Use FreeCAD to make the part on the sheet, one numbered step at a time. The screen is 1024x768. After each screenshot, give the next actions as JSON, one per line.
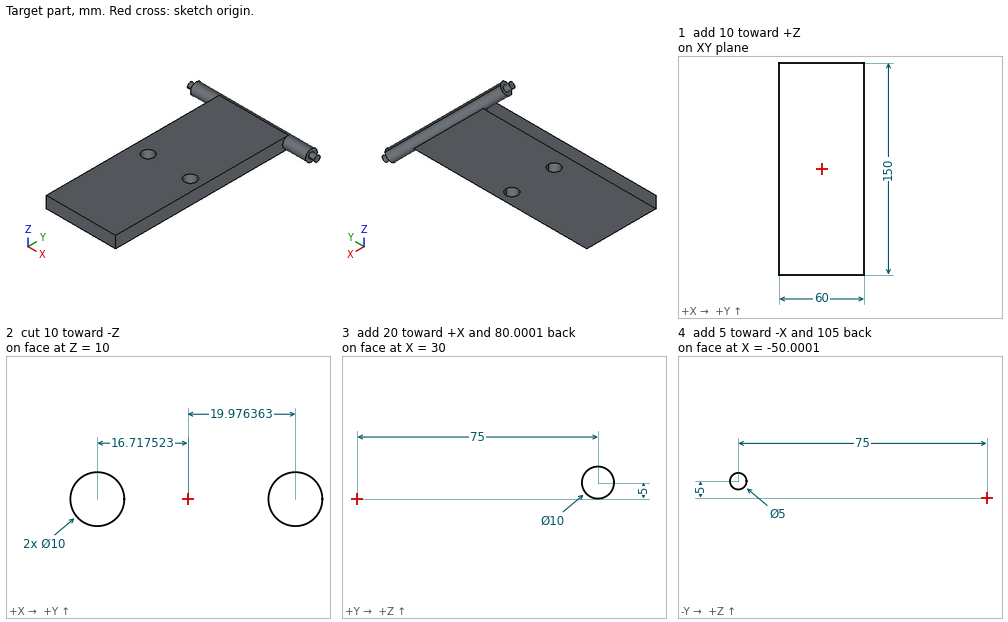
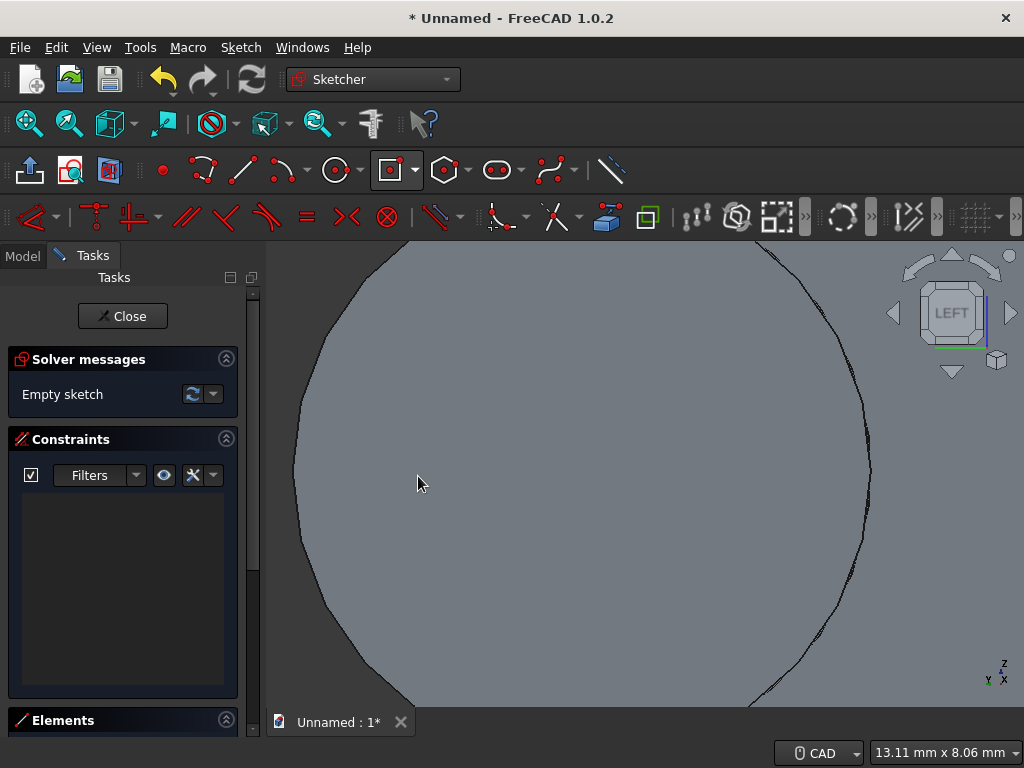
{"action": "left_click", "coordinate": [336, 170]}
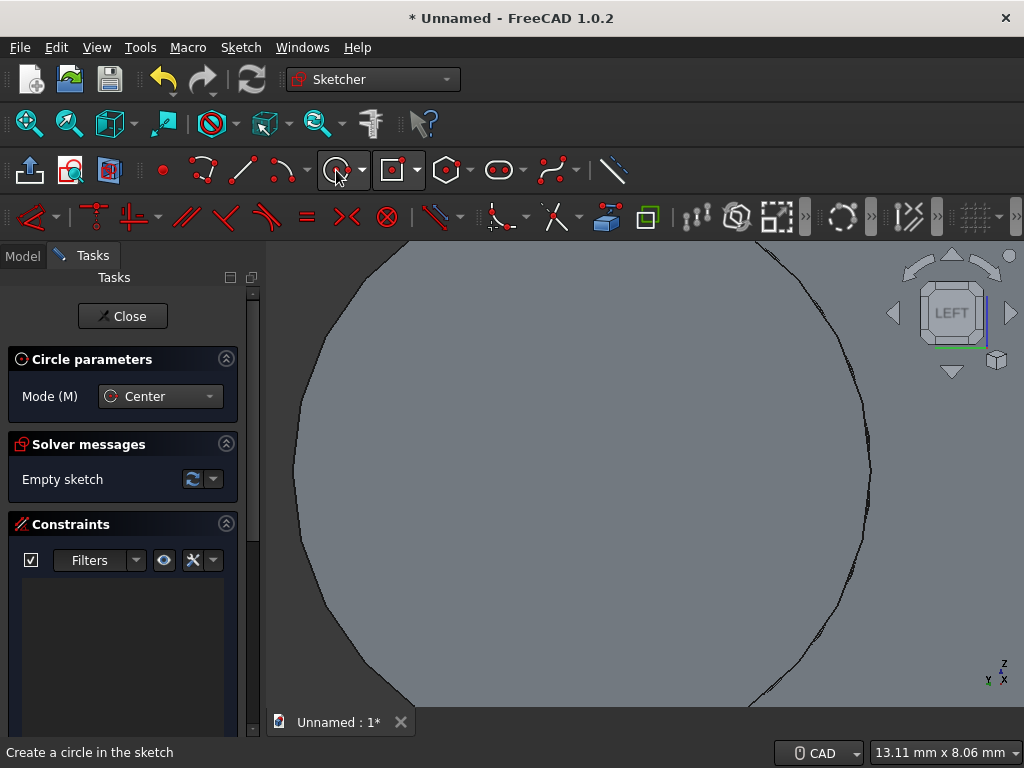
{"action": "left_click", "coordinate": [582, 471]}
{"action": "left_click", "coordinate": [684, 369]}
{"action": "key", "text": "Escape"}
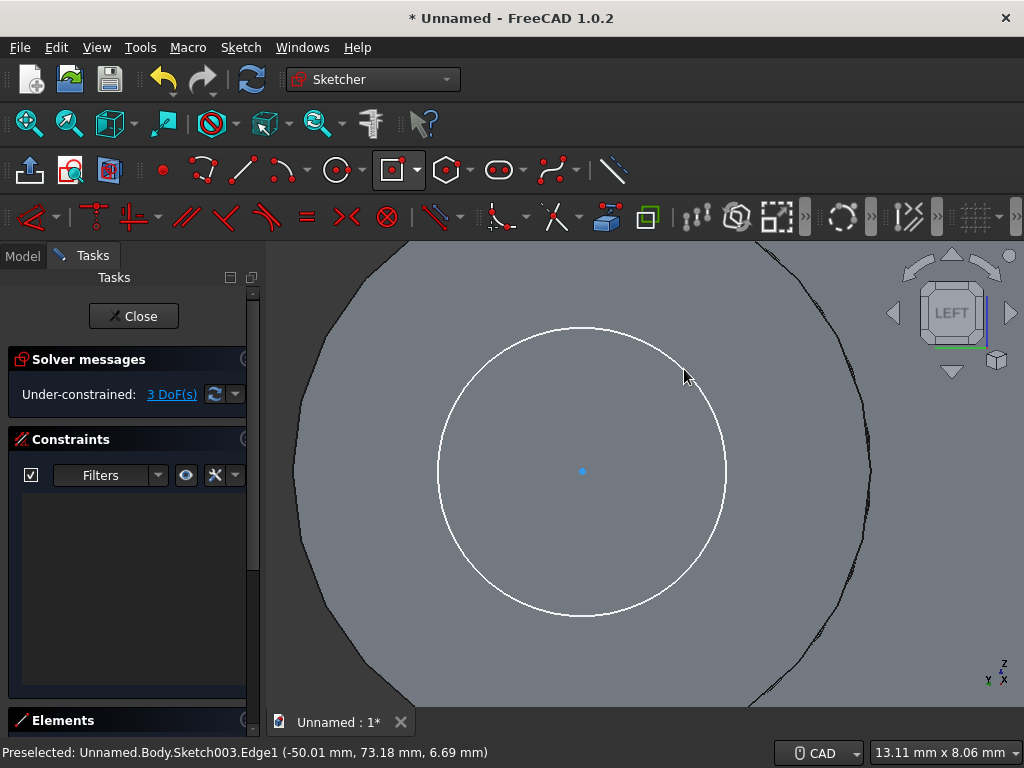
{"action": "left_click", "coordinate": [32, 218]}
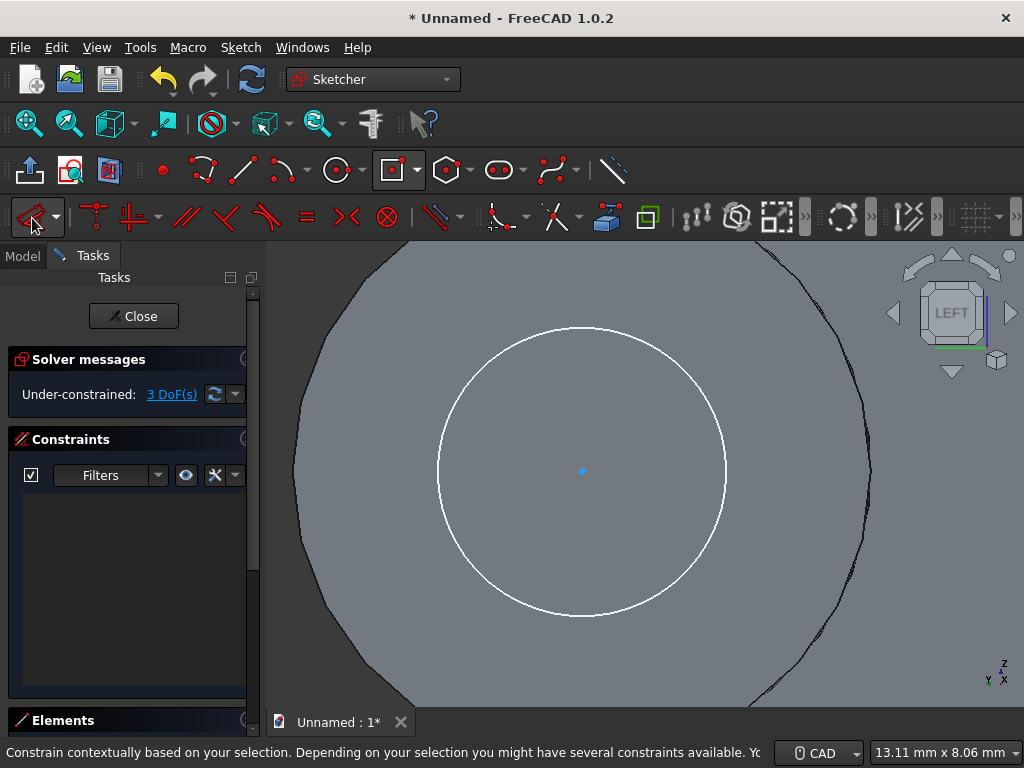
{"action": "left_click", "coordinate": [684, 370]}
{"action": "left_click", "coordinate": [707, 347]}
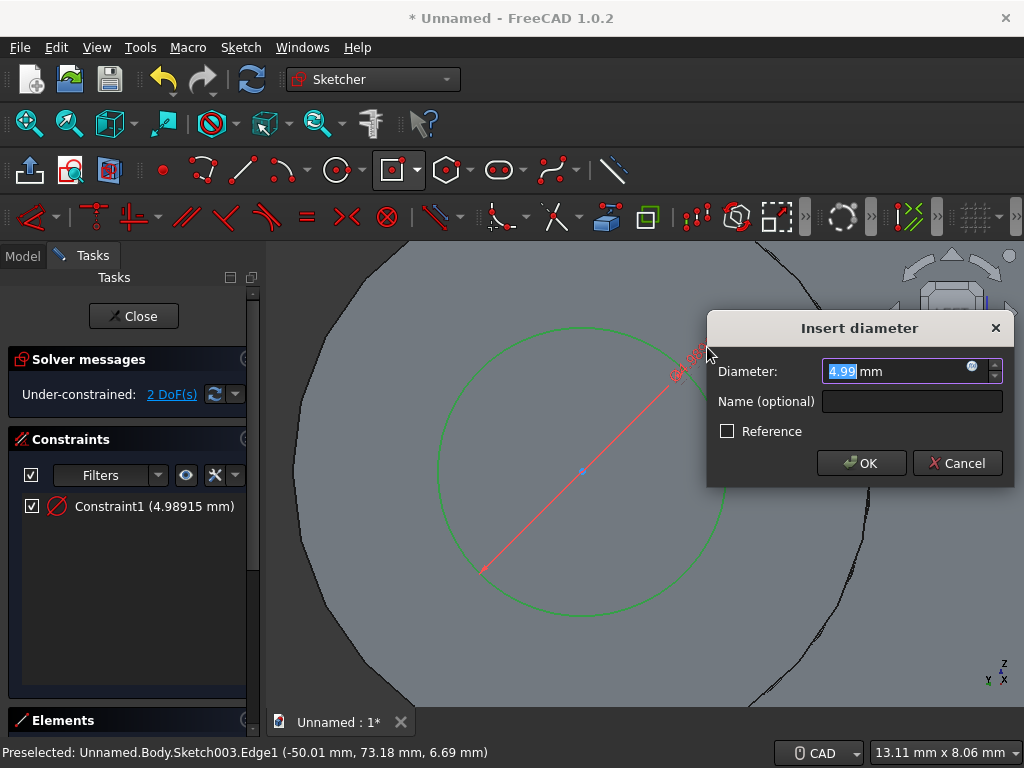
{"action": "type", "text": "5"}
{"action": "key", "text": "Return"}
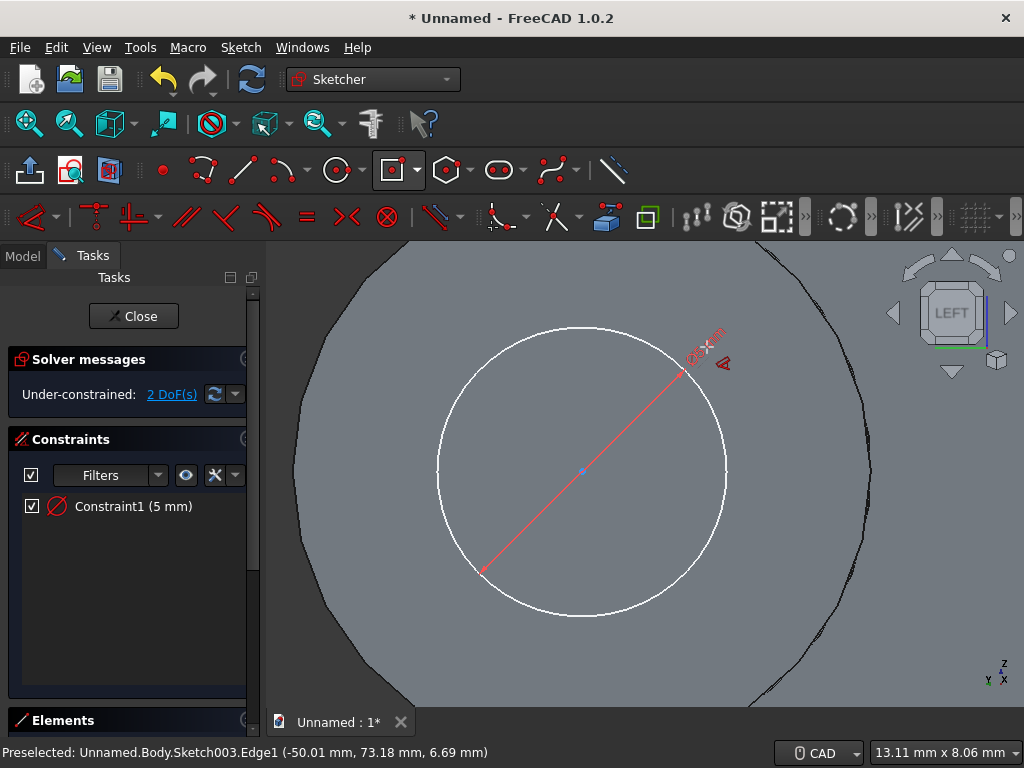
{"action": "left_click", "coordinate": [582, 472]}
{"action": "left_click", "coordinate": [548, 575]}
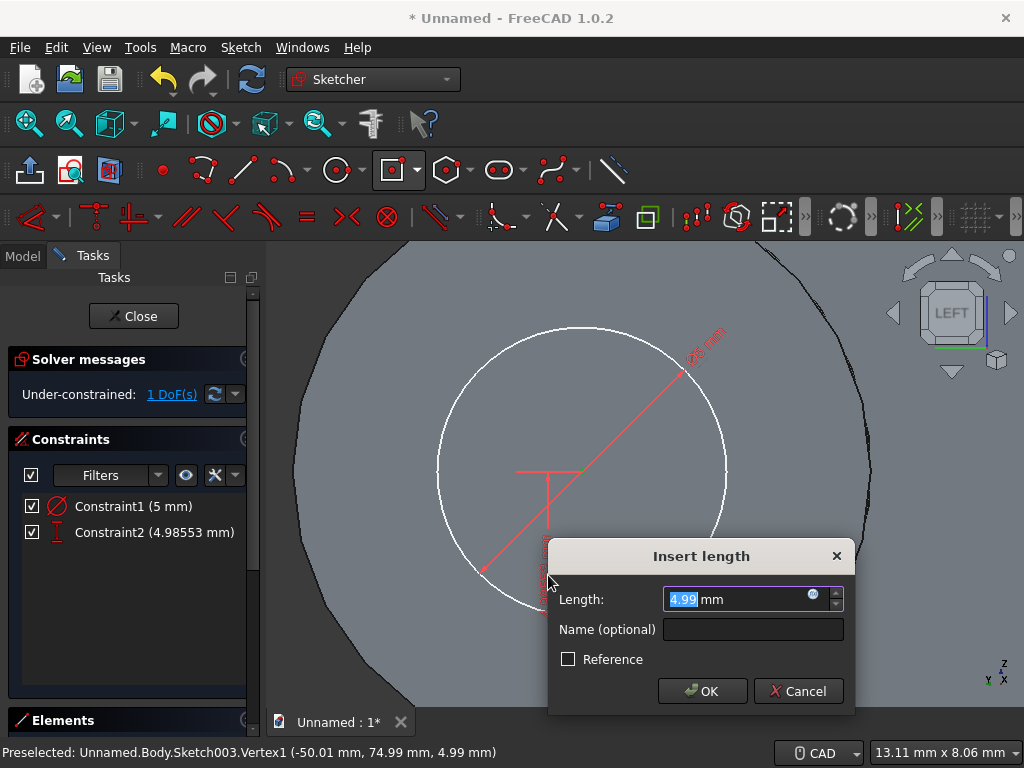
{"action": "type", "text": "5"}
{"action": "key", "text": "Return"}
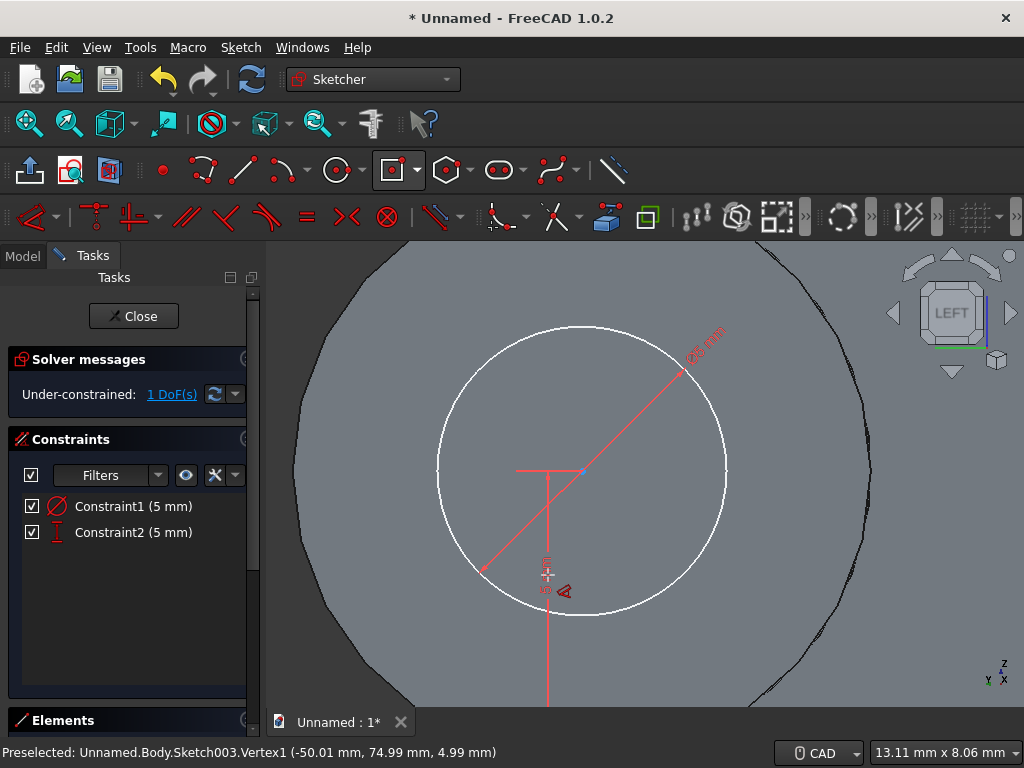
{"action": "left_click", "coordinate": [582, 471]}
{"action": "left_click", "coordinate": [657, 437]}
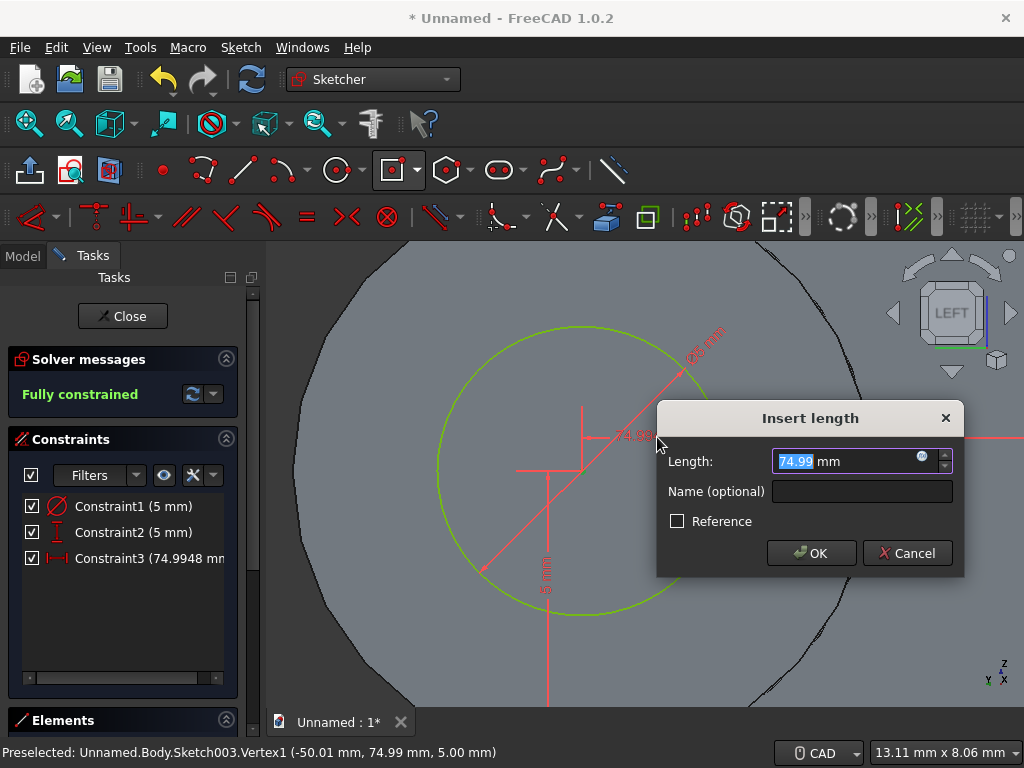
{"action": "type", "text": "75"}
{"action": "key", "text": "Return"}
{"action": "key", "text": "Escape"}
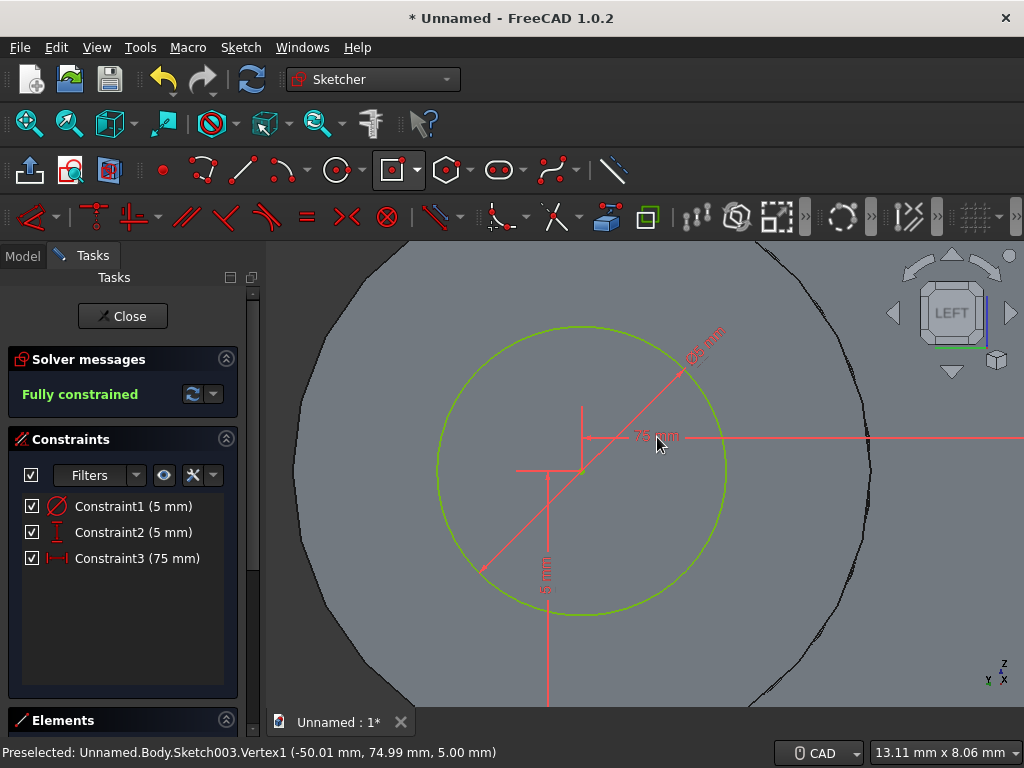
{"action": "left_click", "coordinate": [123, 316]}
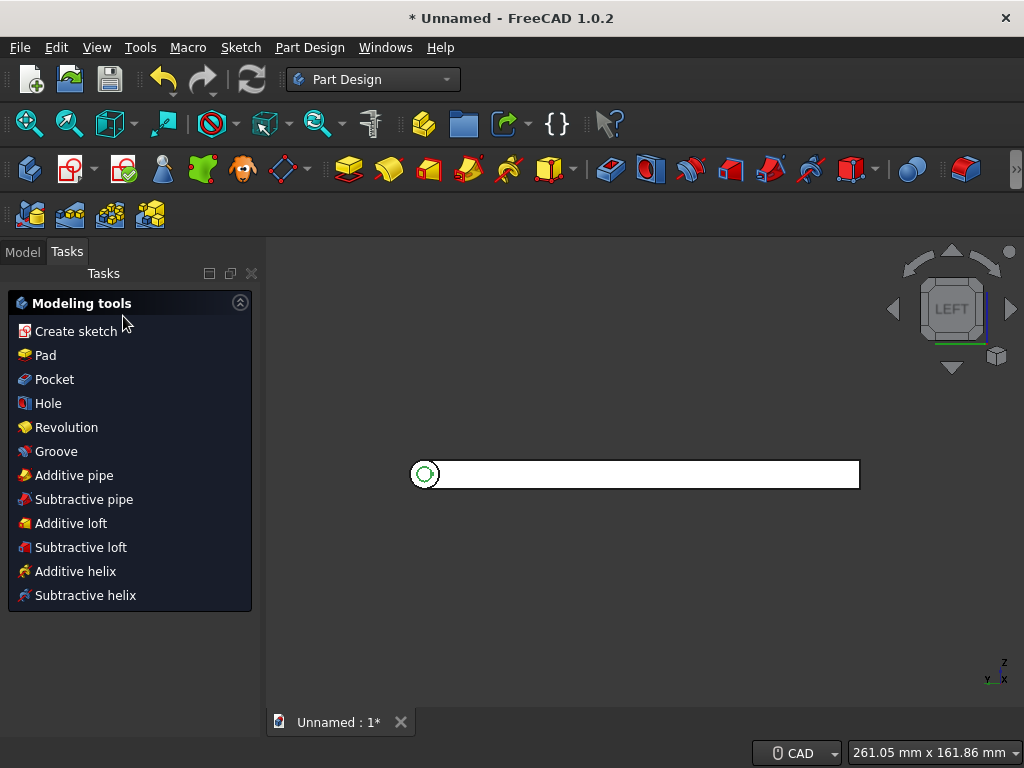
{"action": "left_click", "coordinate": [350, 170]}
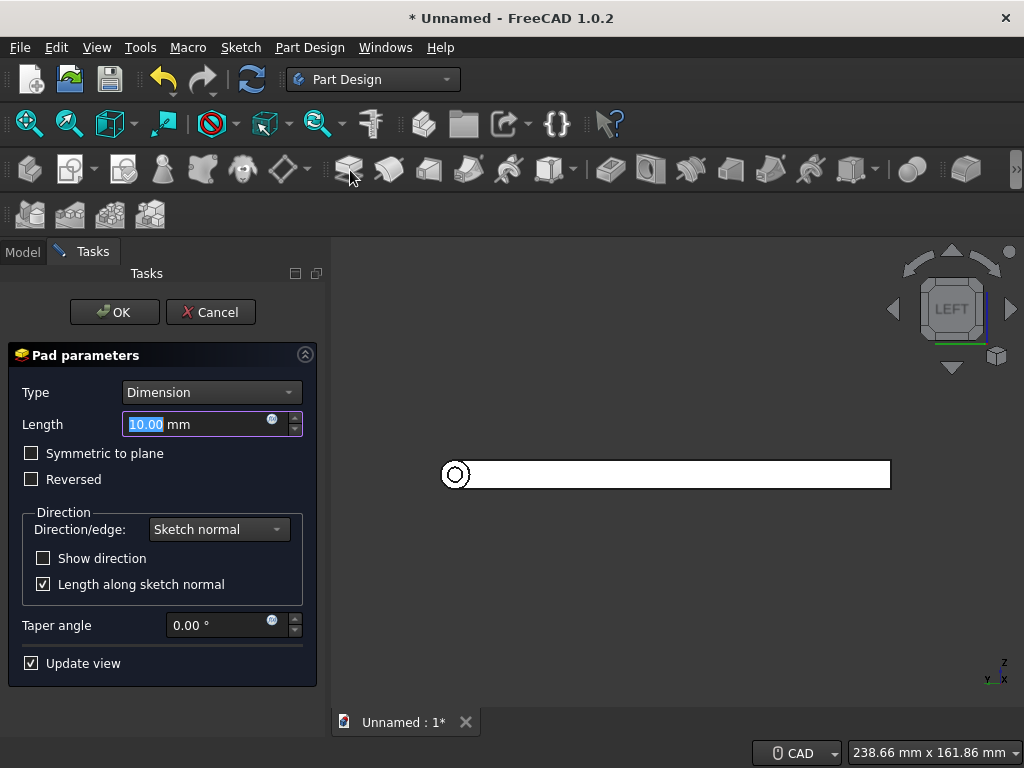
{"action": "left_click", "coordinate": [212, 392]}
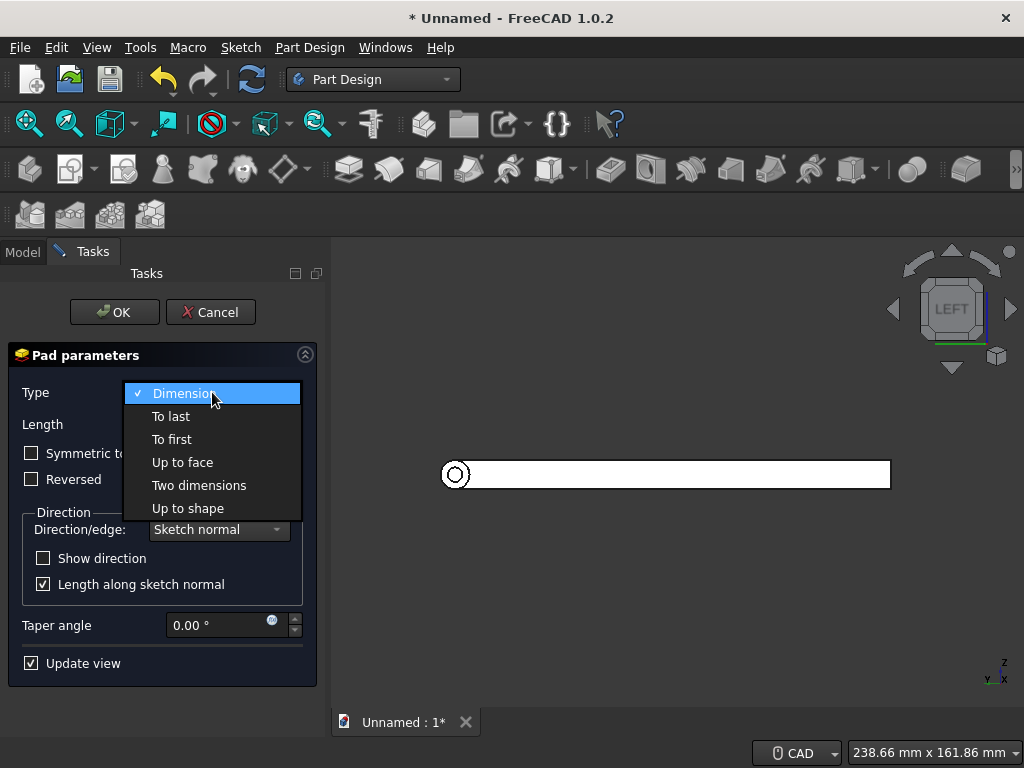
{"action": "left_click", "coordinate": [212, 486]}